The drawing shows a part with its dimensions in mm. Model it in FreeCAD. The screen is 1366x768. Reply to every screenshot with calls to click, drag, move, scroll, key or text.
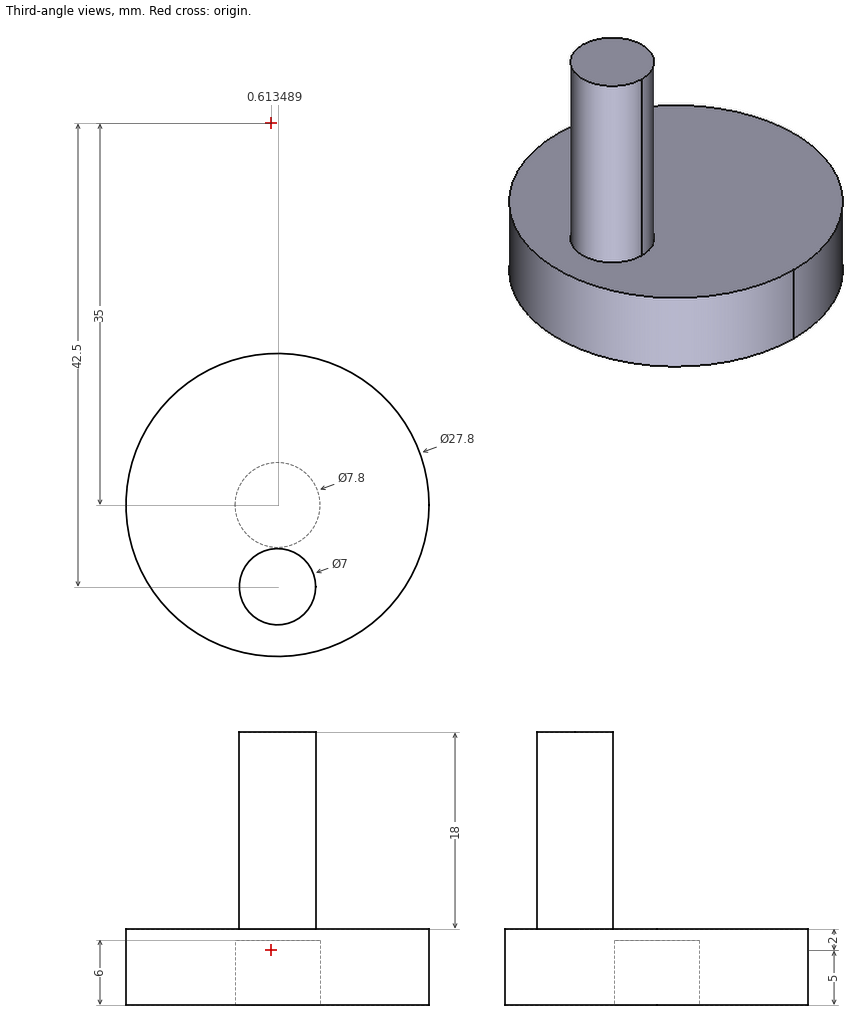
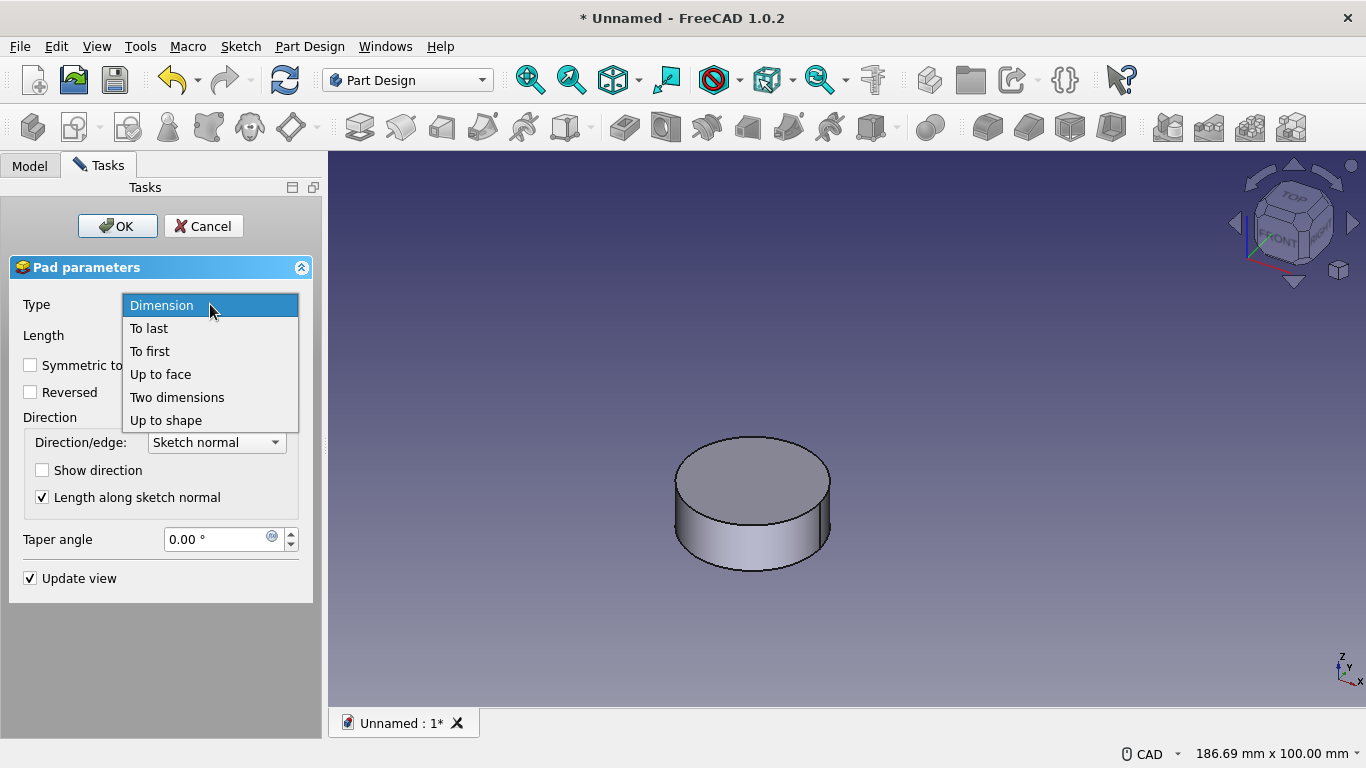
click(208, 398)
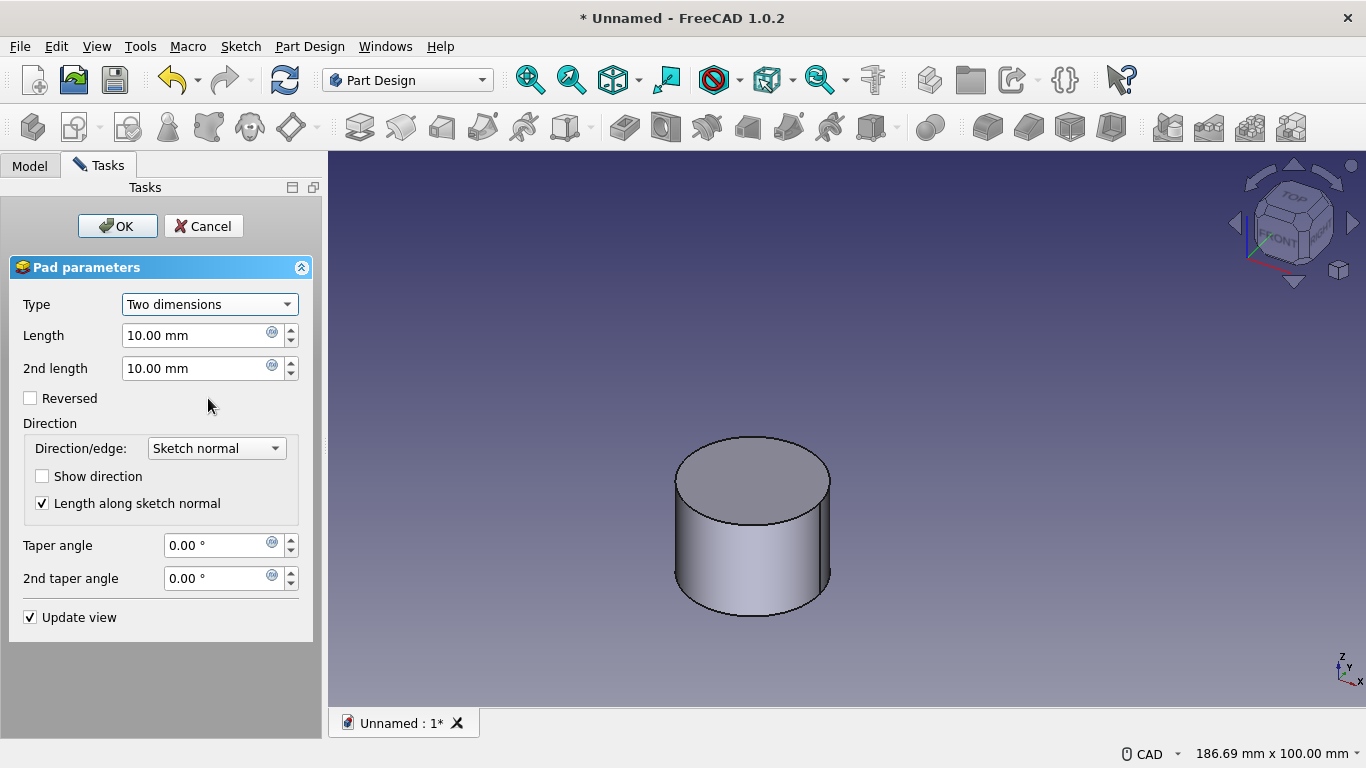
triple_click(204, 336)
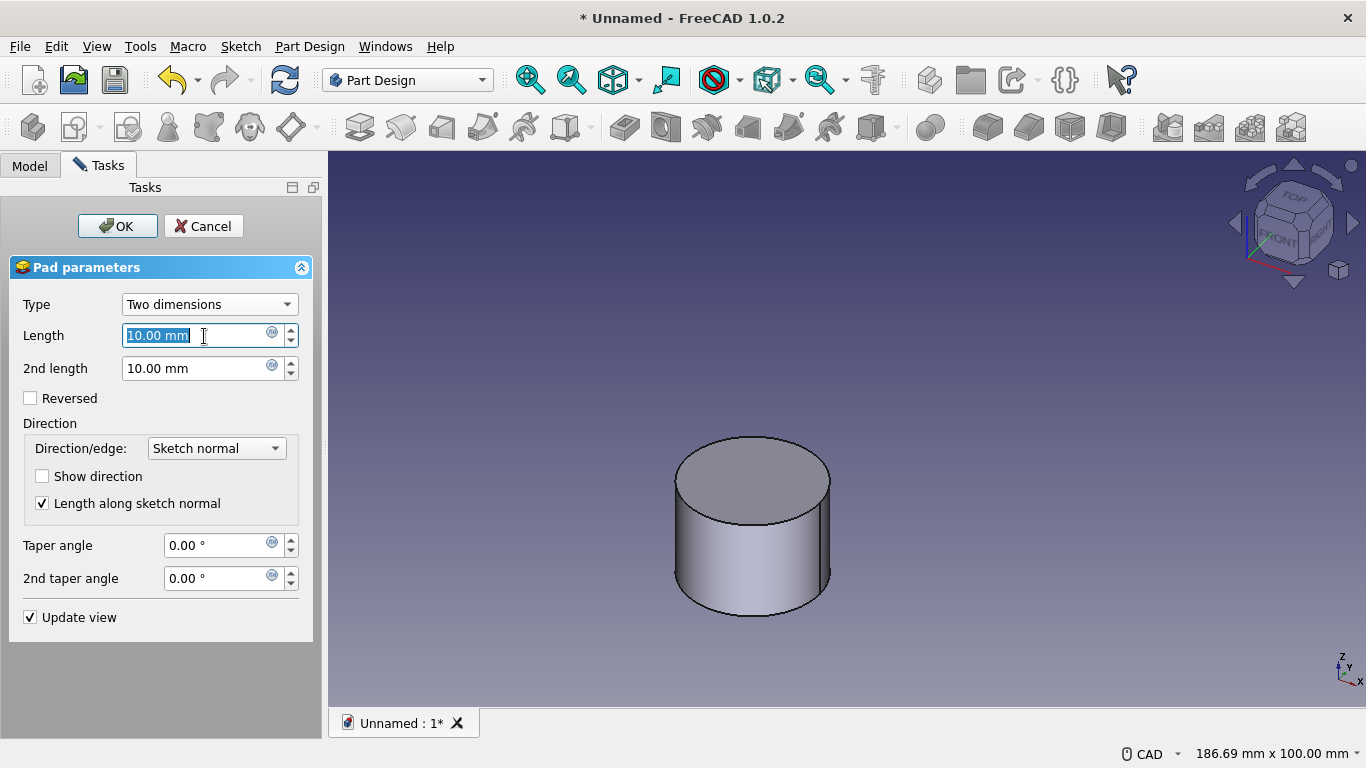
text(2)
key(Tab)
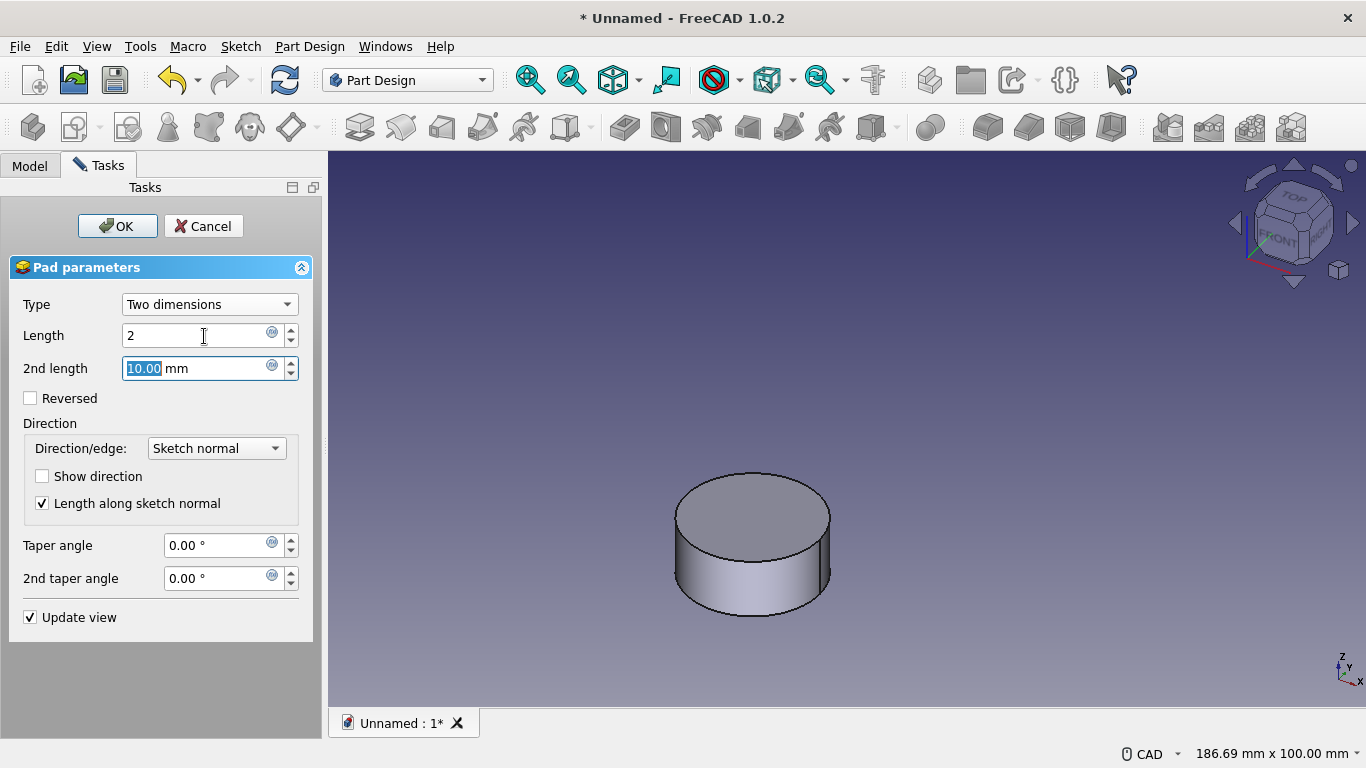
text(5)
key(Tab)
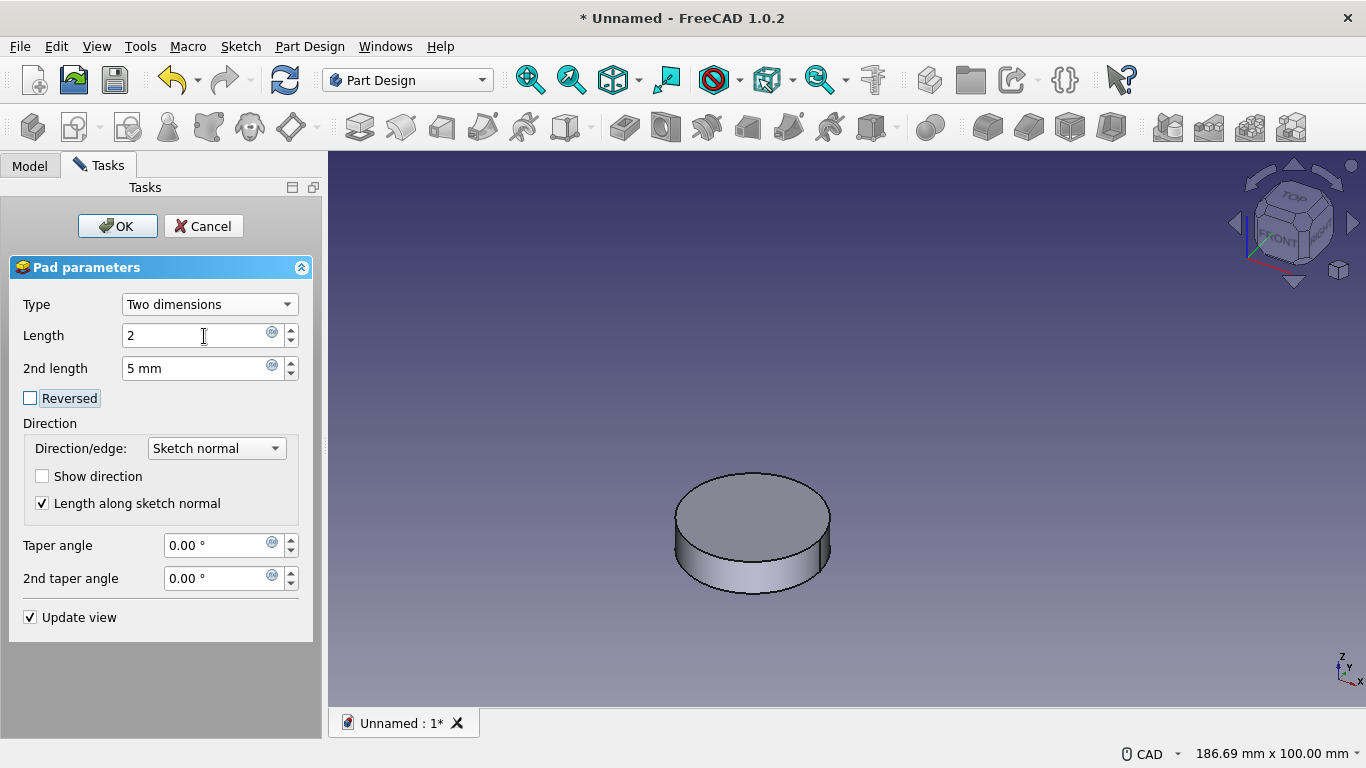
click(118, 226)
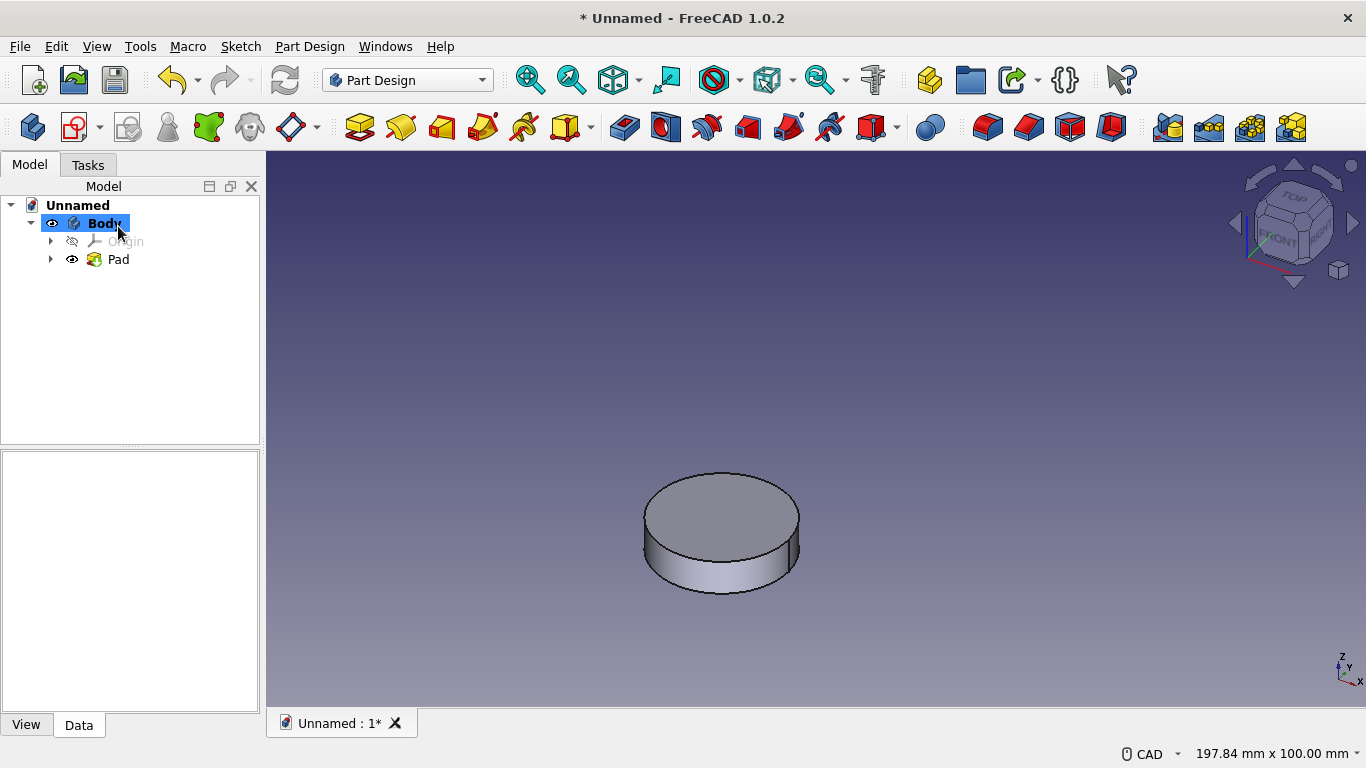
click(531, 80)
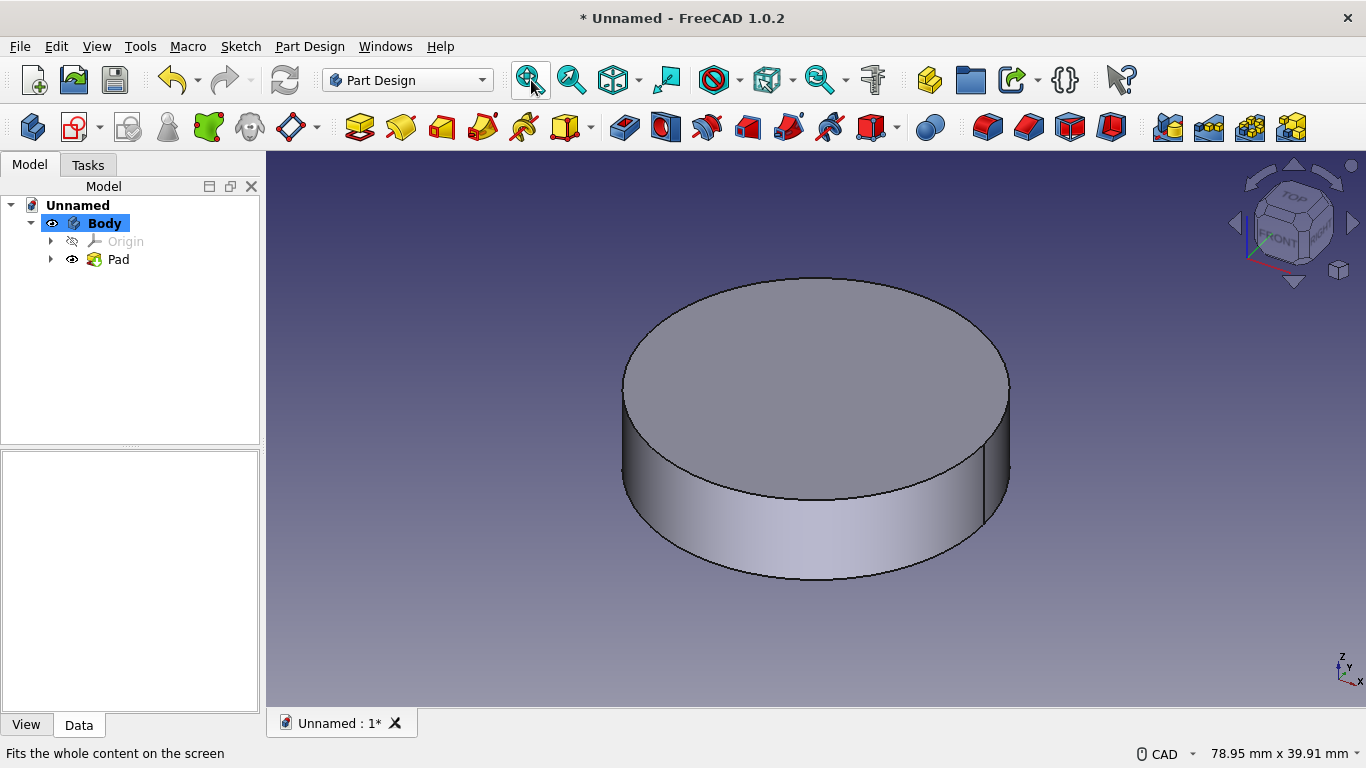
key(5)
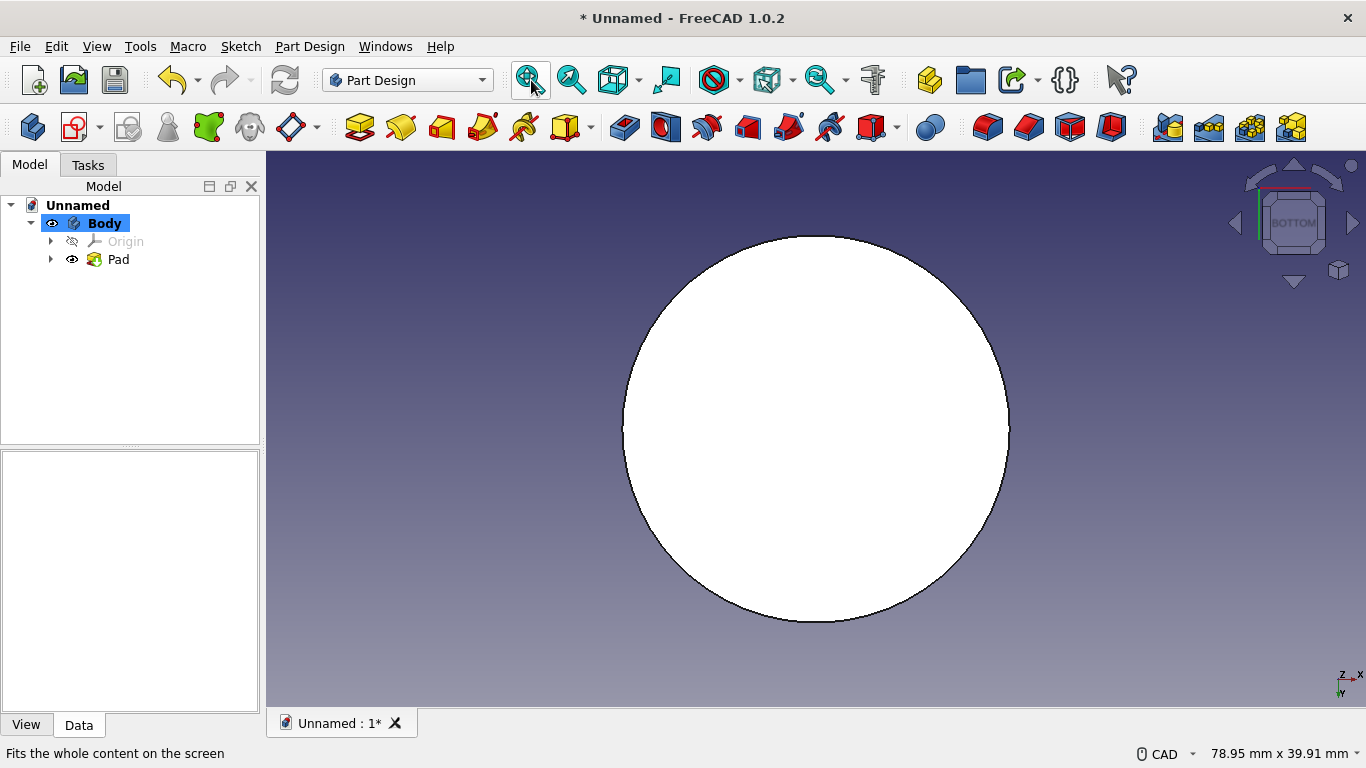
click(816, 428)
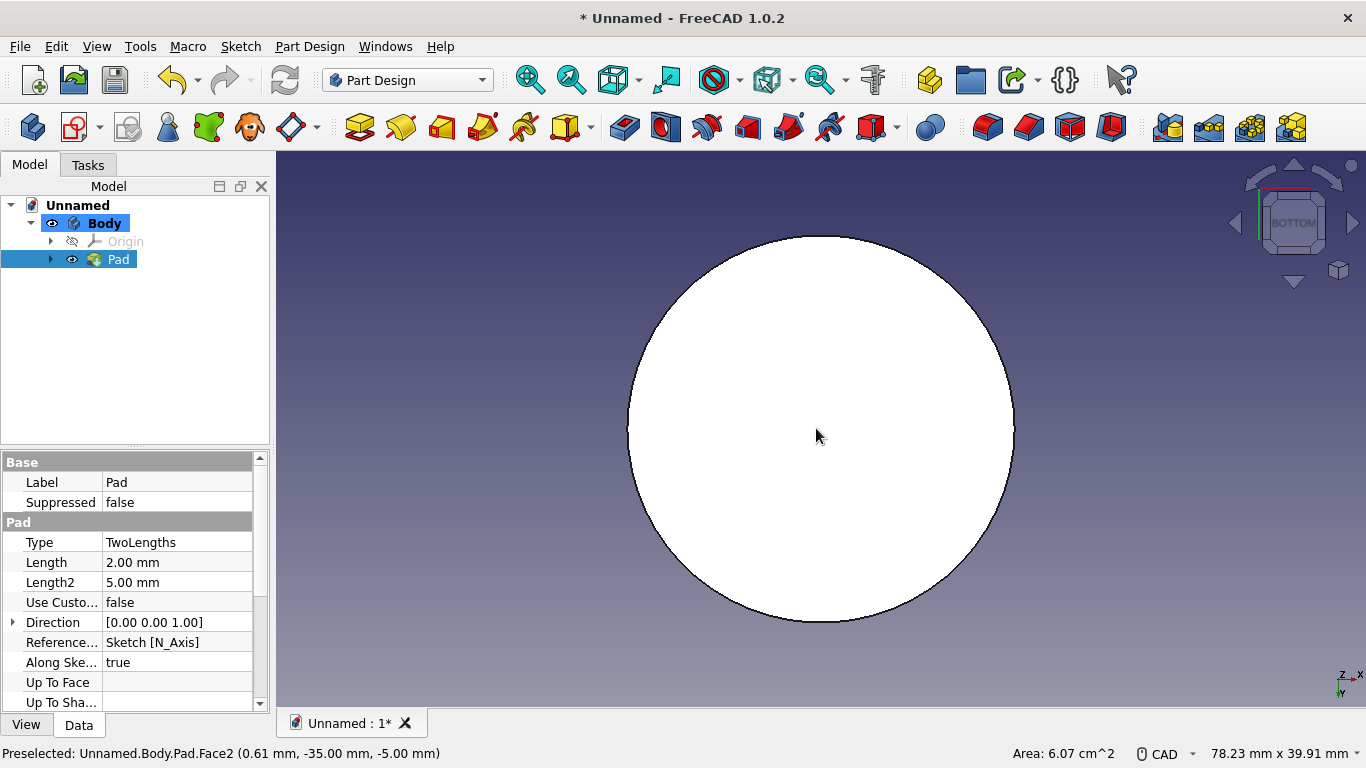
click(74, 128)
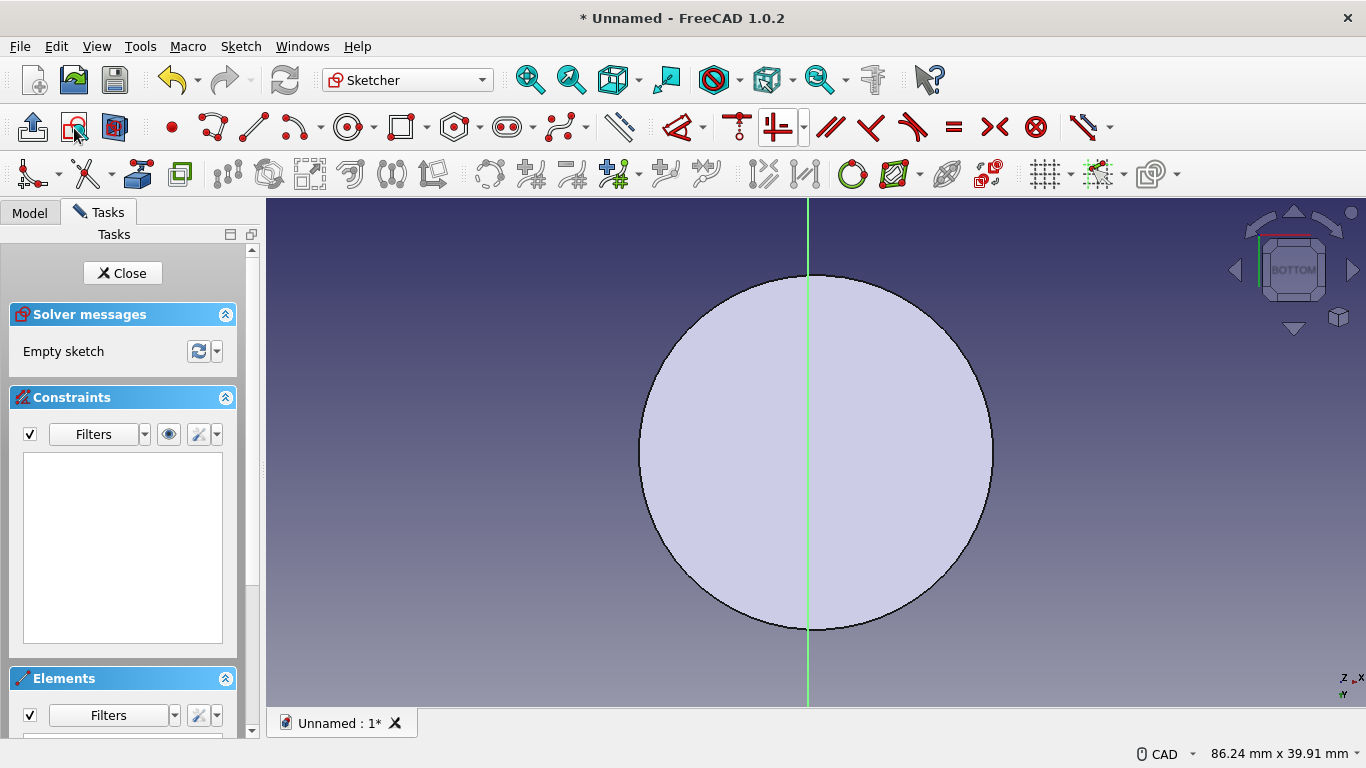
scroll(846, 452, up, 6)